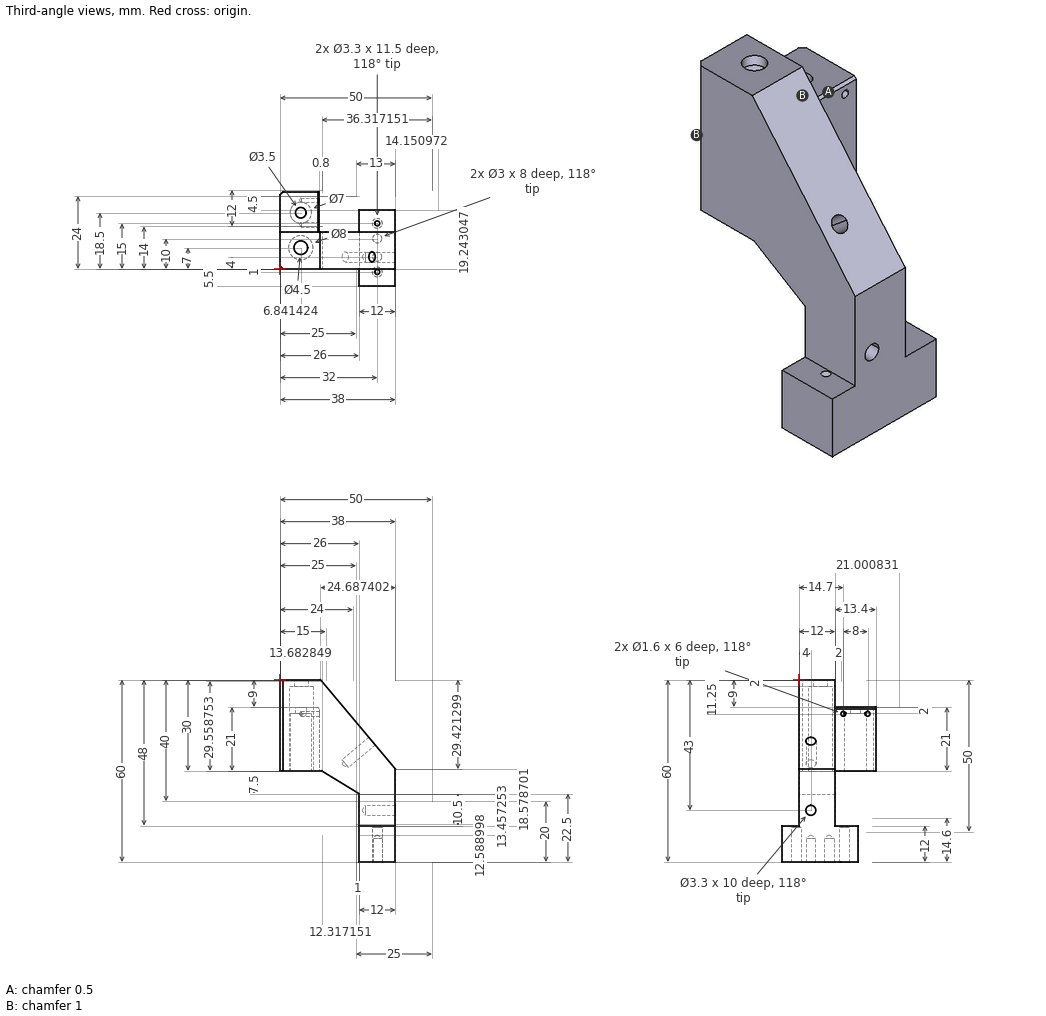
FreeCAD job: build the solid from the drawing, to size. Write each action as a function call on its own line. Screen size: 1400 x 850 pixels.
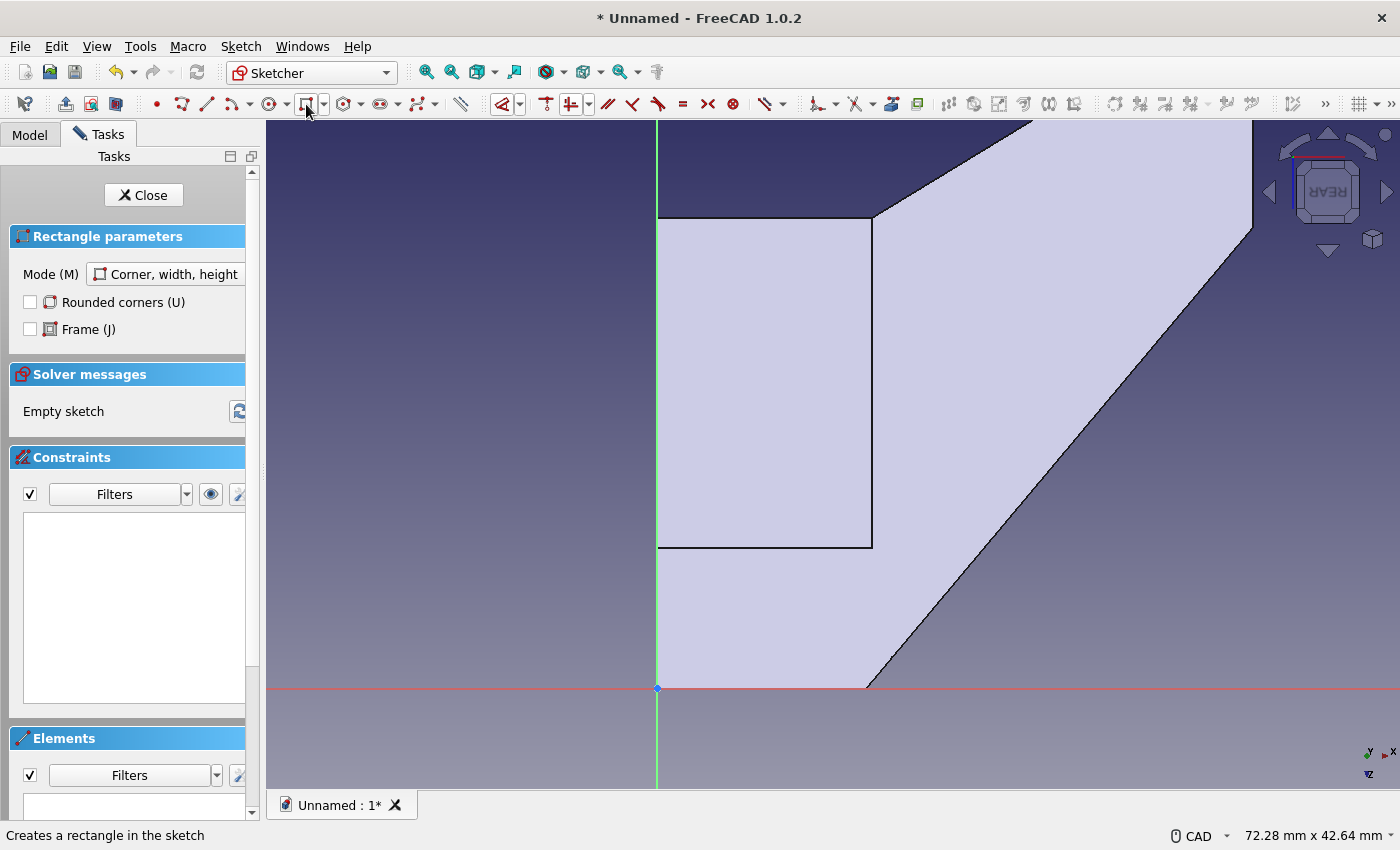
click(657, 218)
click(872, 548)
key(Escape)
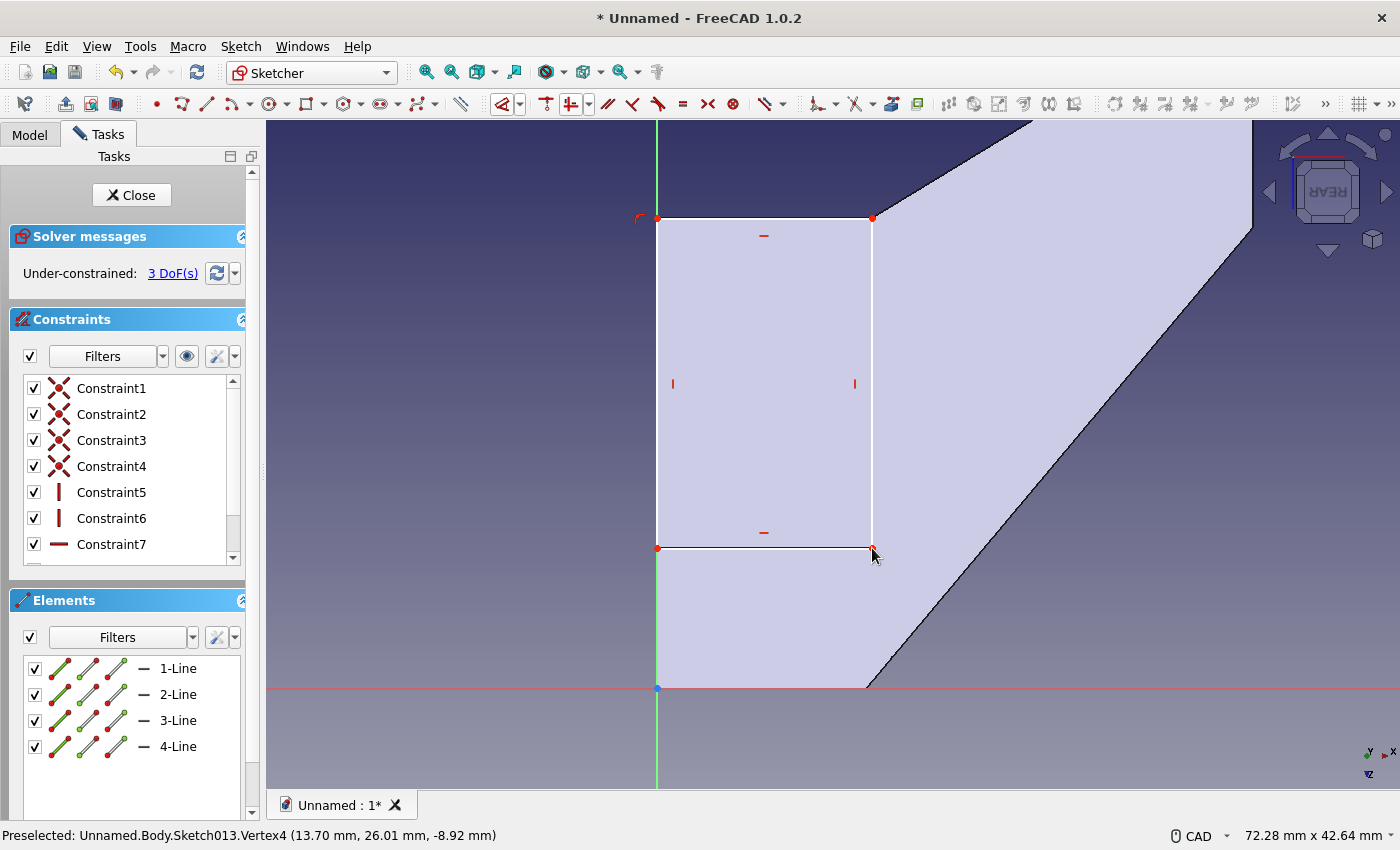
click(657, 318)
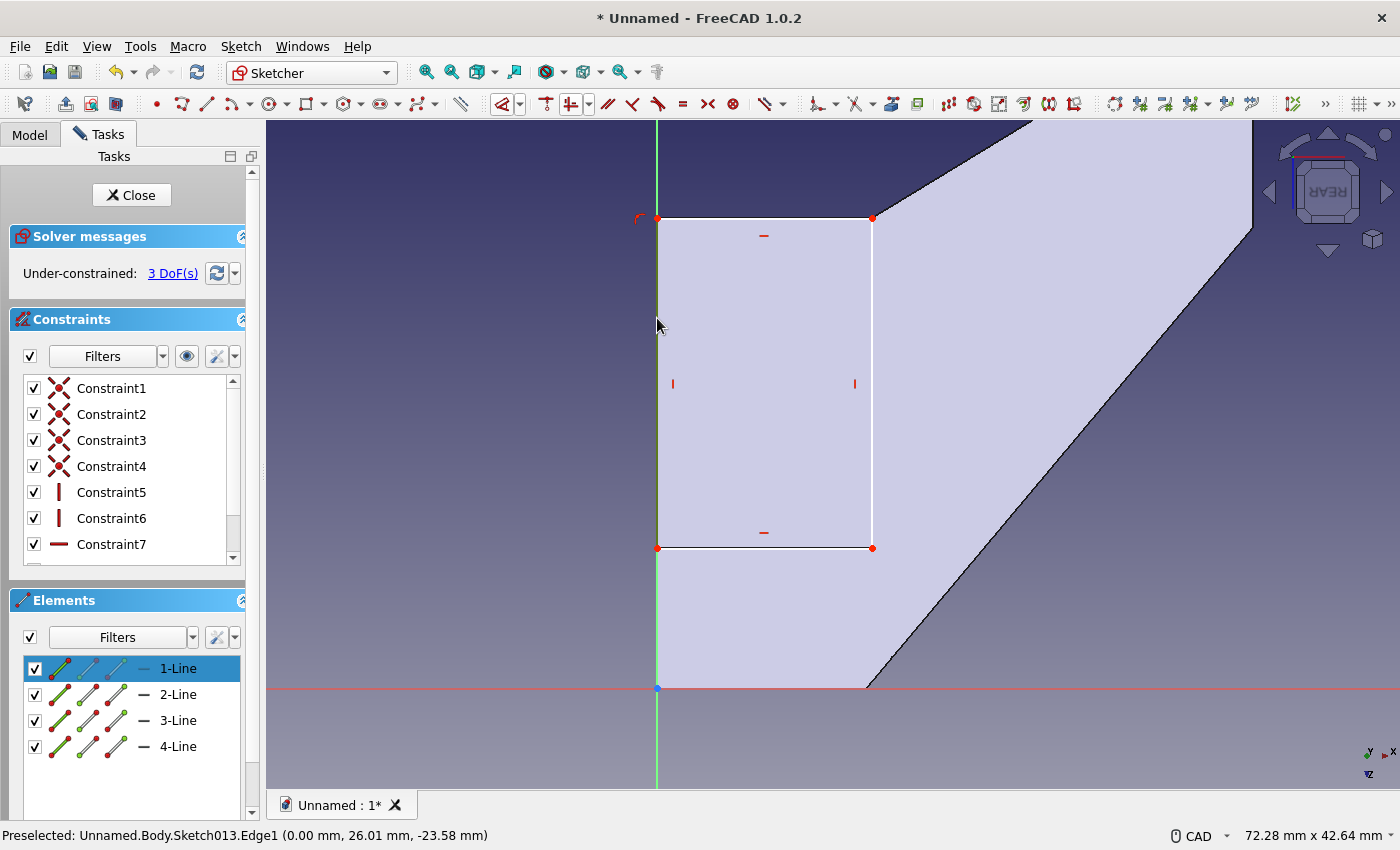
key(i)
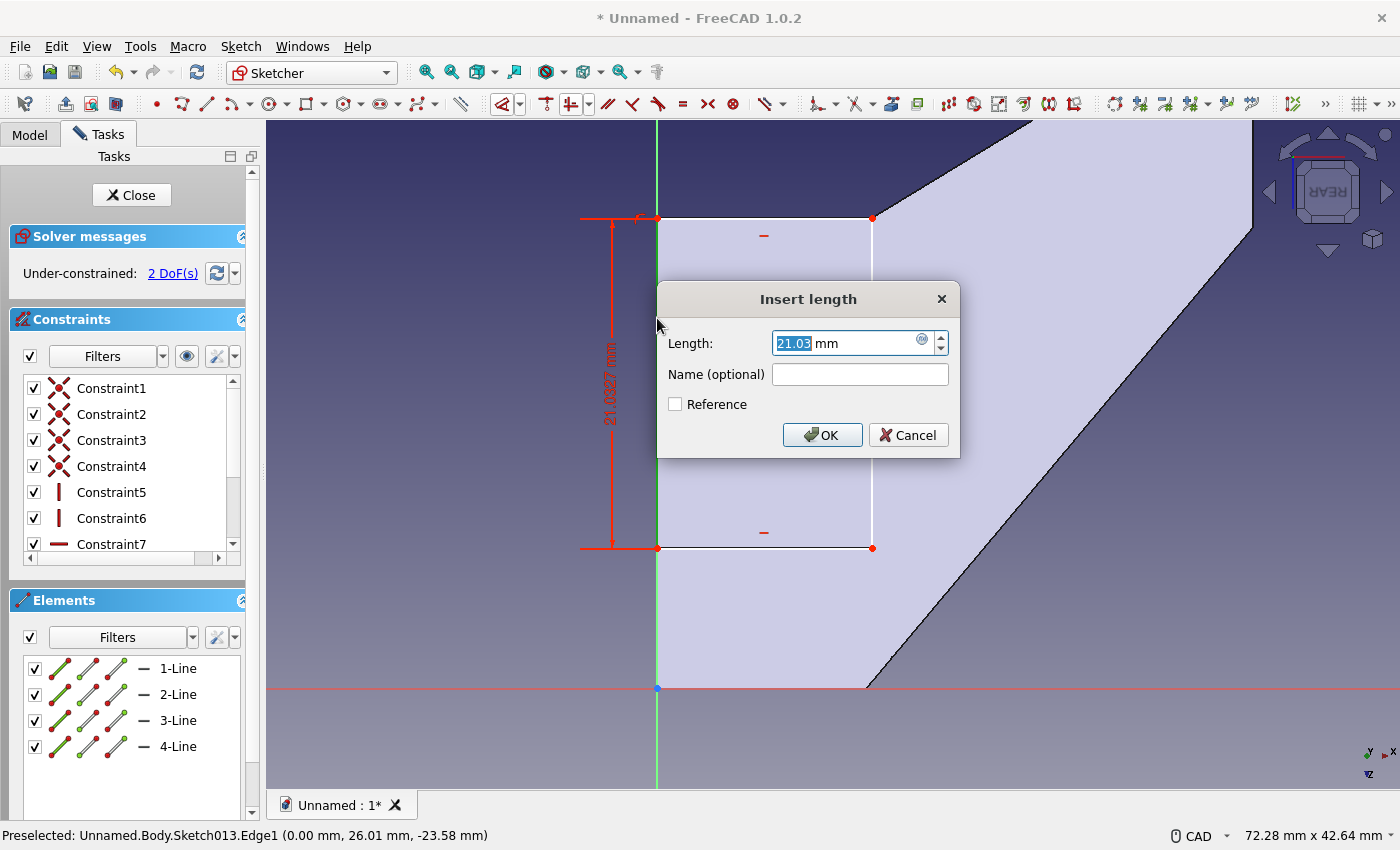
text(21)
key(Return)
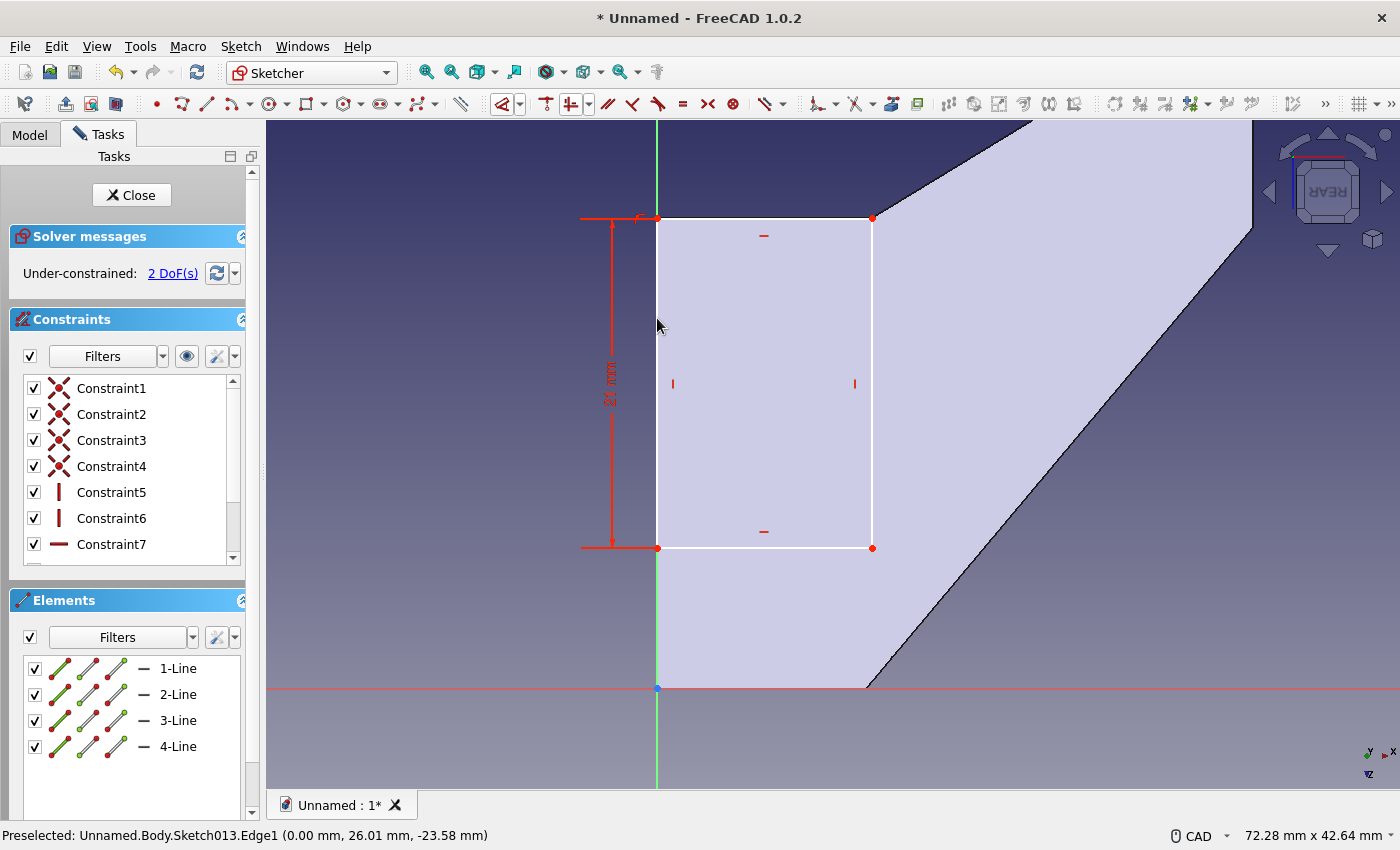
click(657, 548)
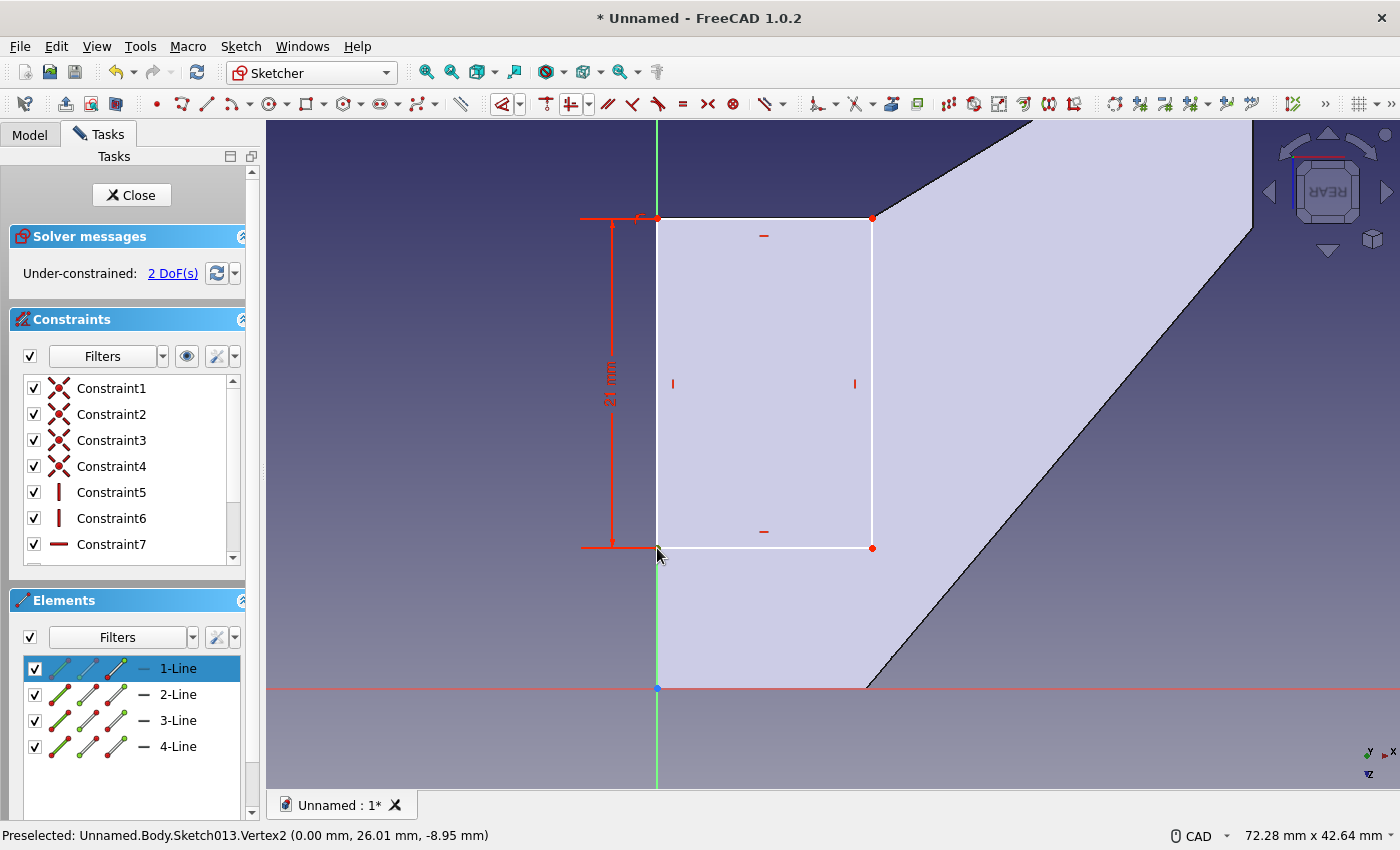
key(i)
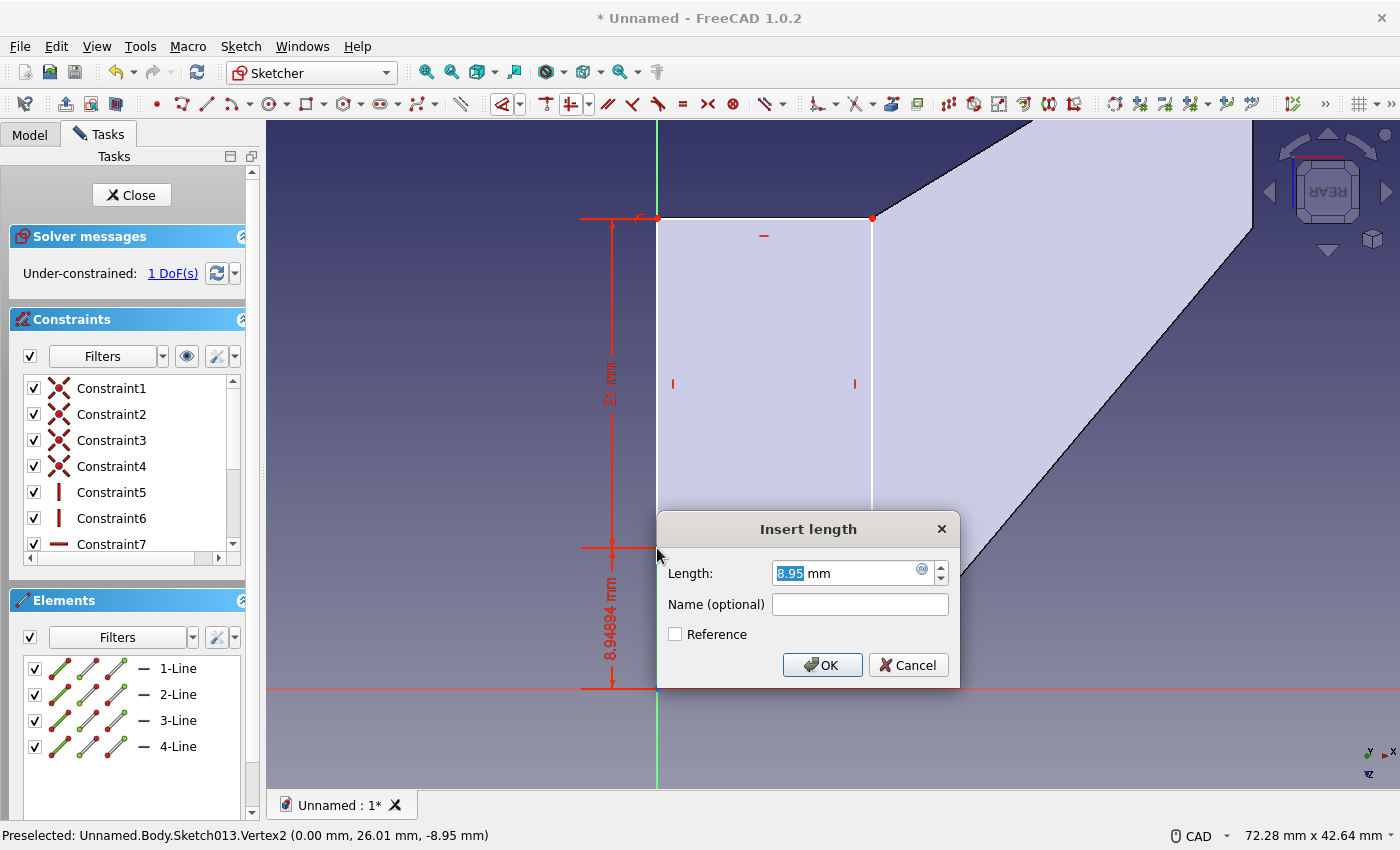
text(9)
key(Return)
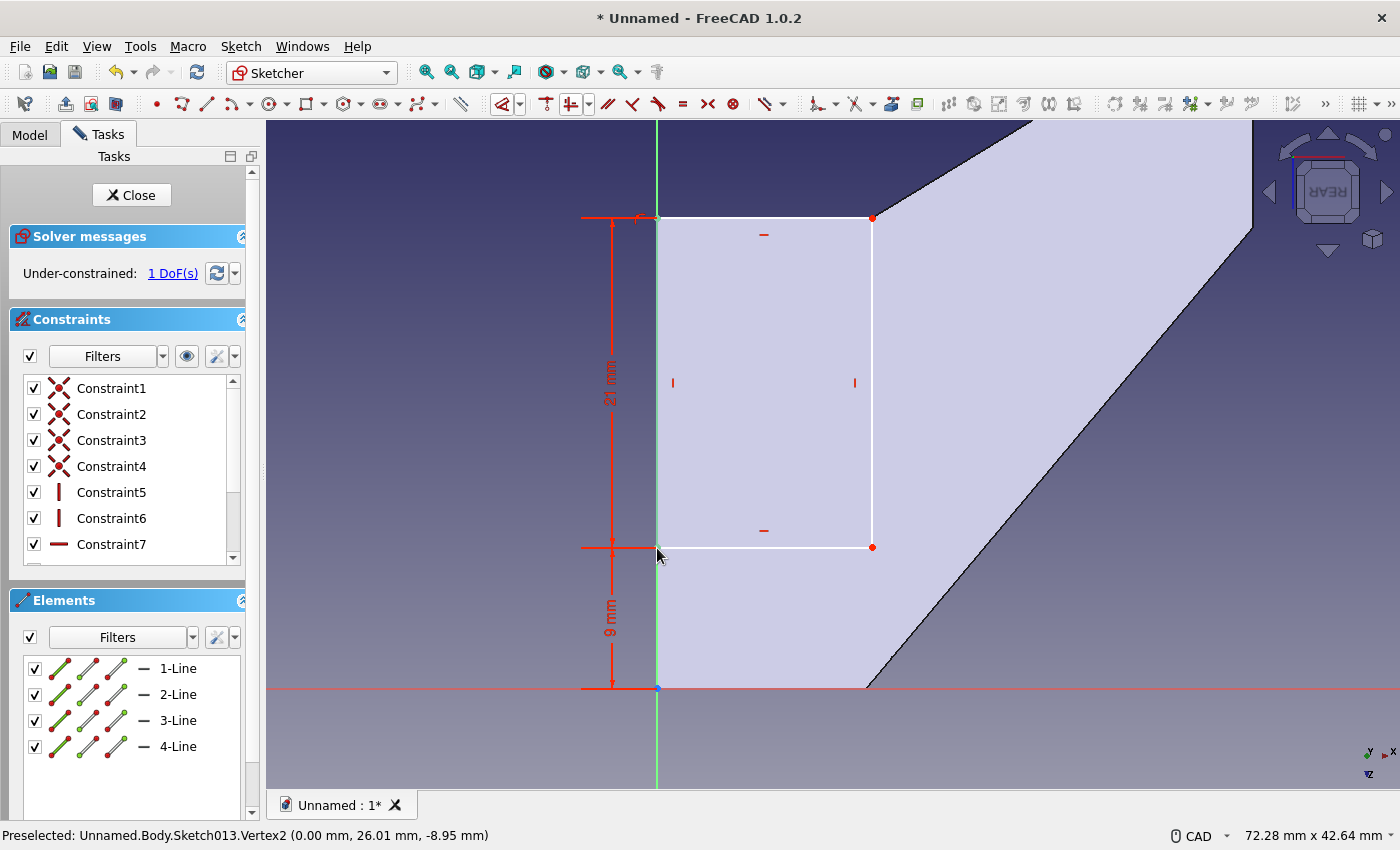
click(722, 548)